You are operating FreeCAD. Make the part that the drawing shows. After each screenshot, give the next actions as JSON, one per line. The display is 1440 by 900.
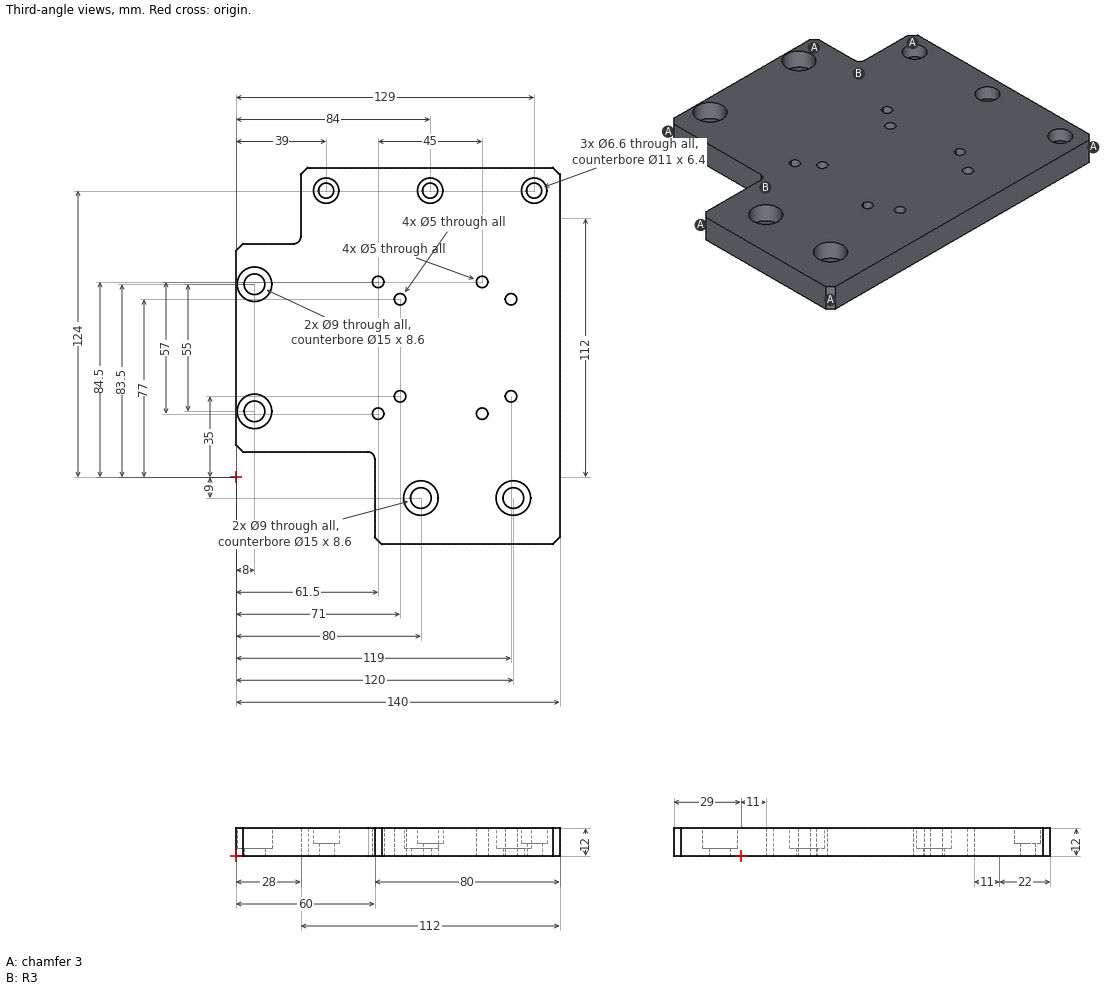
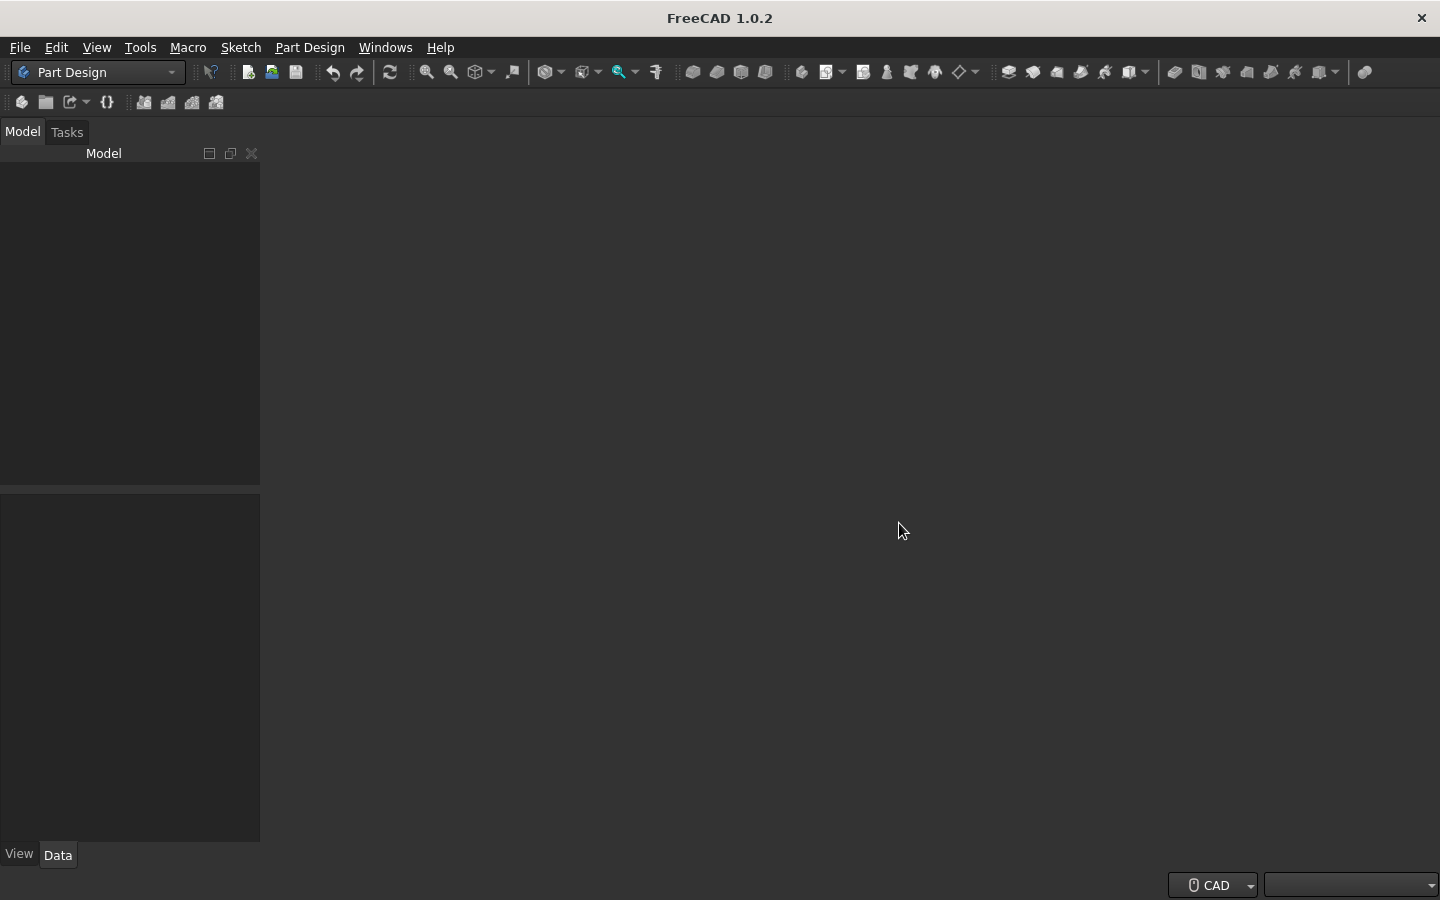
{"action": "left_click", "coordinate": [248, 72]}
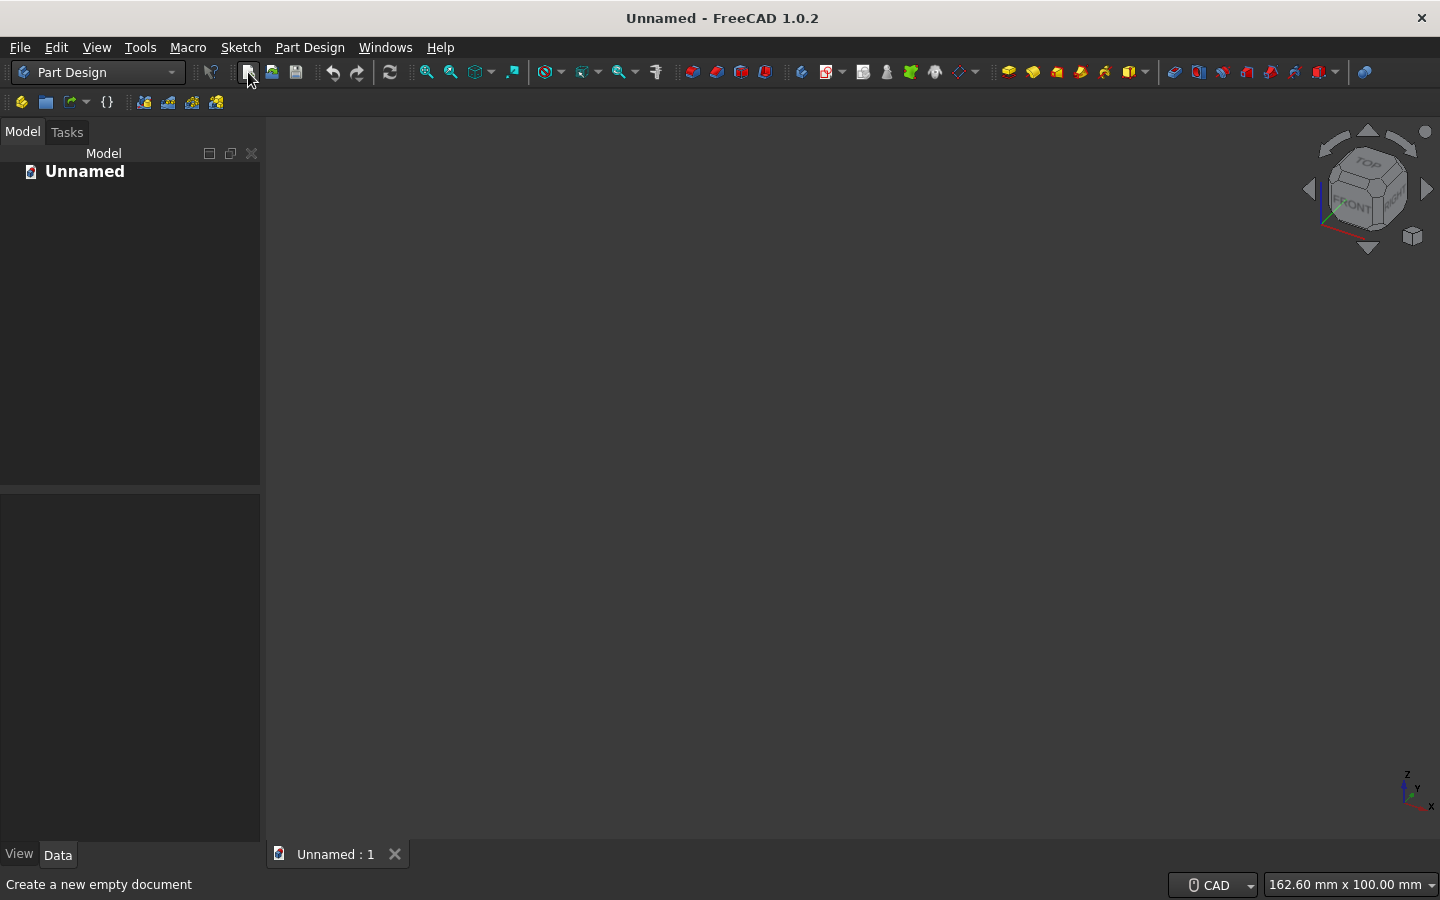
{"action": "left_click", "coordinate": [826, 72]}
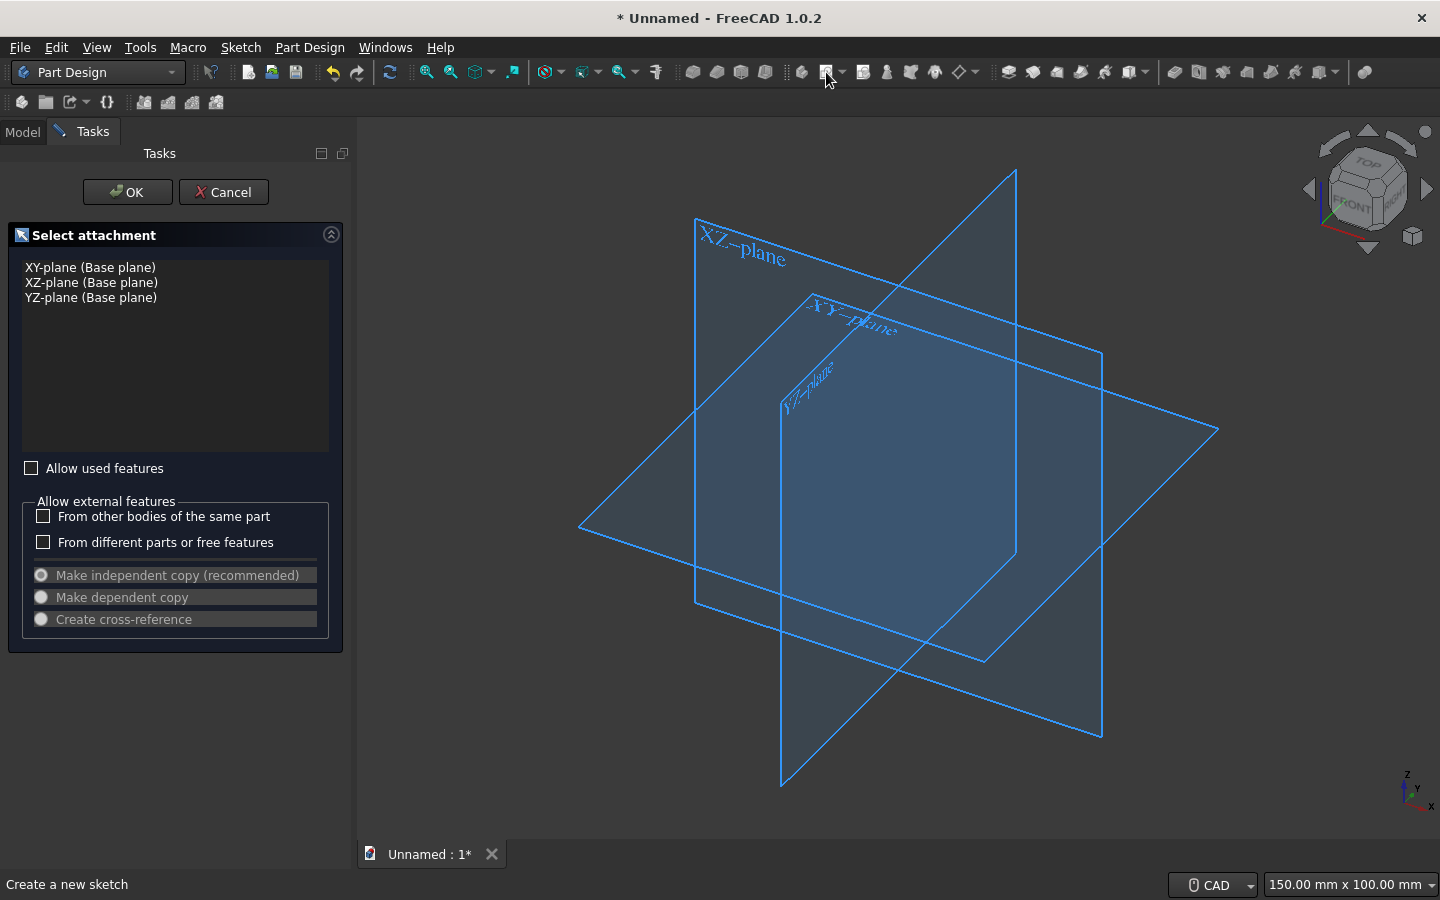
{"action": "left_click", "coordinate": [82, 268]}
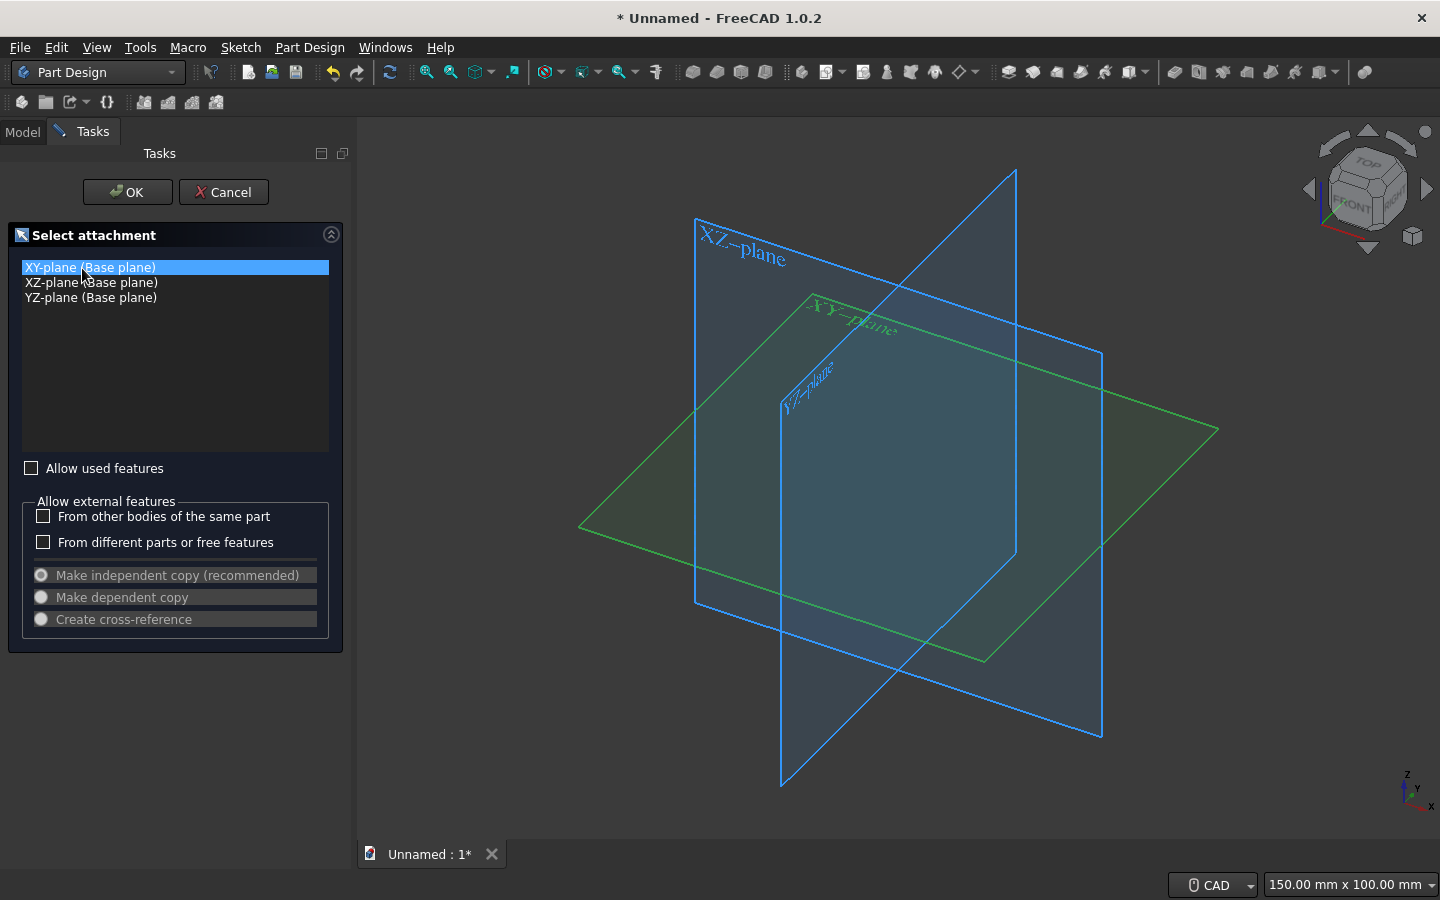
{"action": "left_click", "coordinate": [128, 192]}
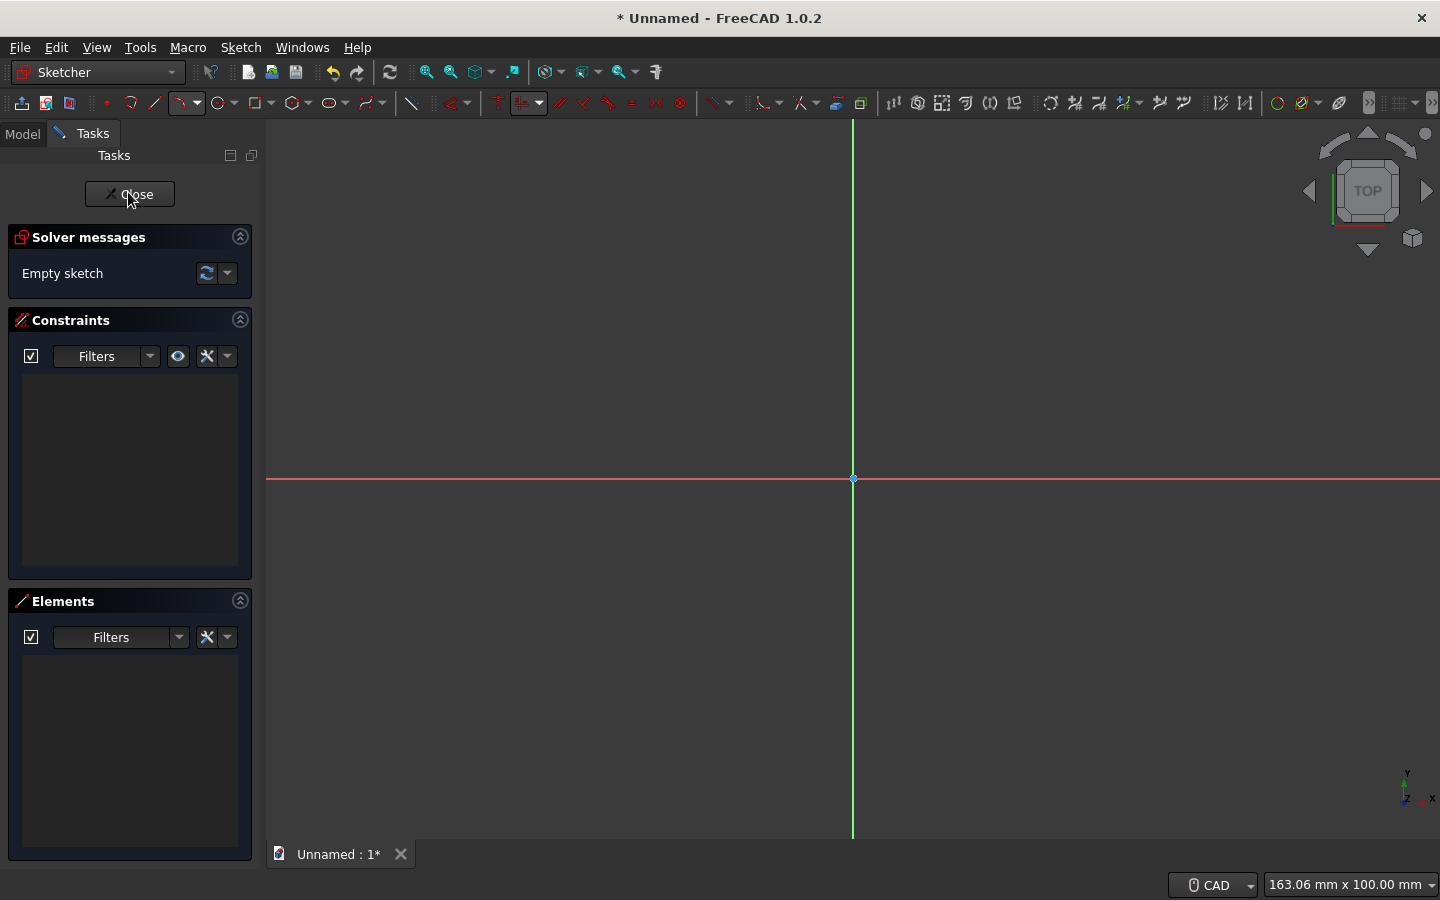
{"action": "scroll", "coordinate": [294, 811], "scroll_direction": "down", "scroll_amount": 3}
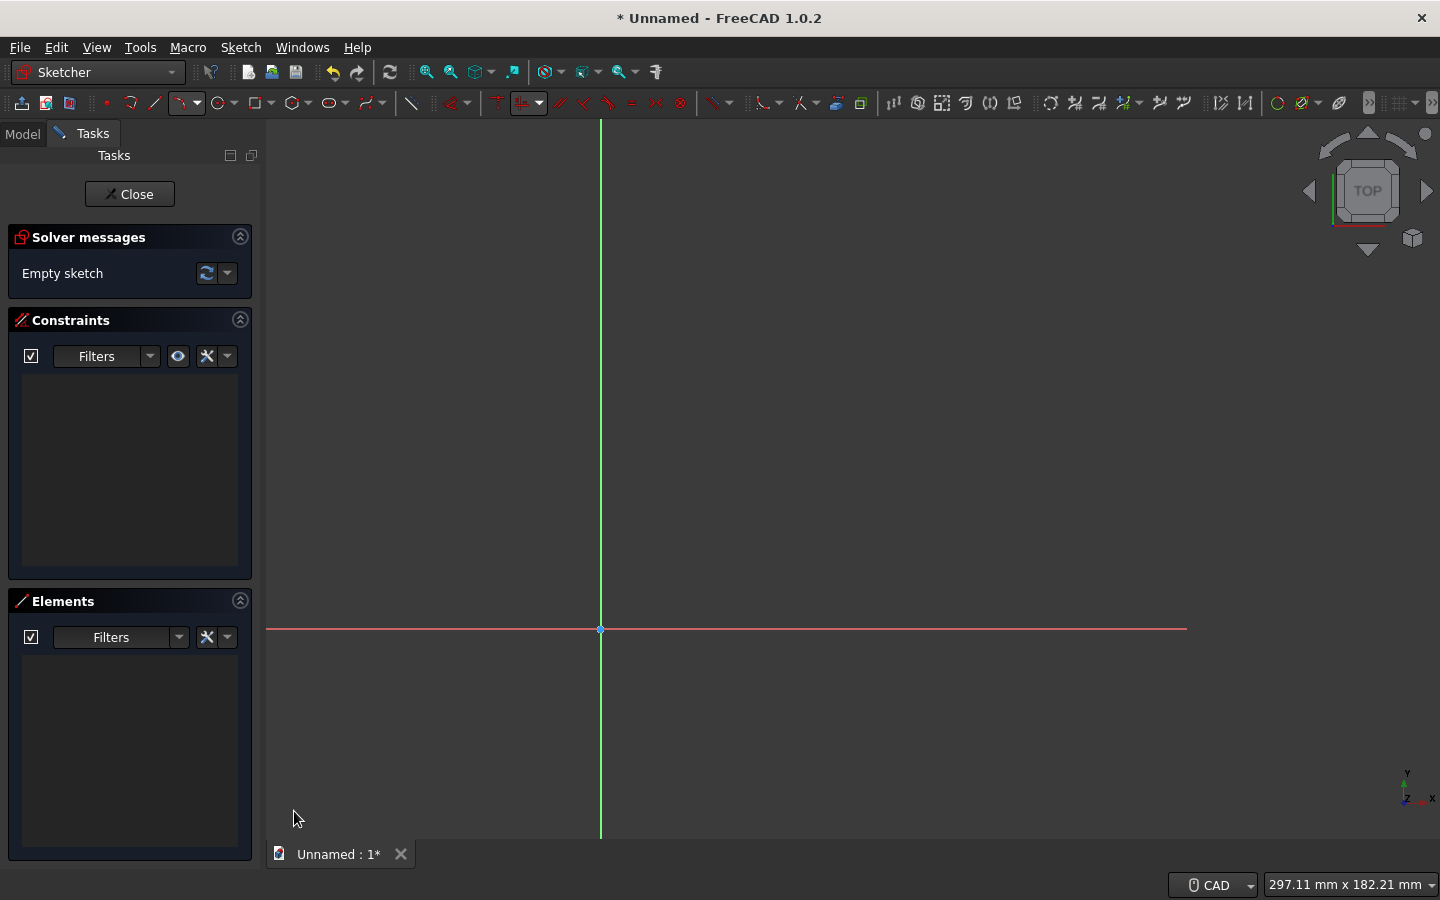
{"action": "left_click", "coordinate": [256, 104]}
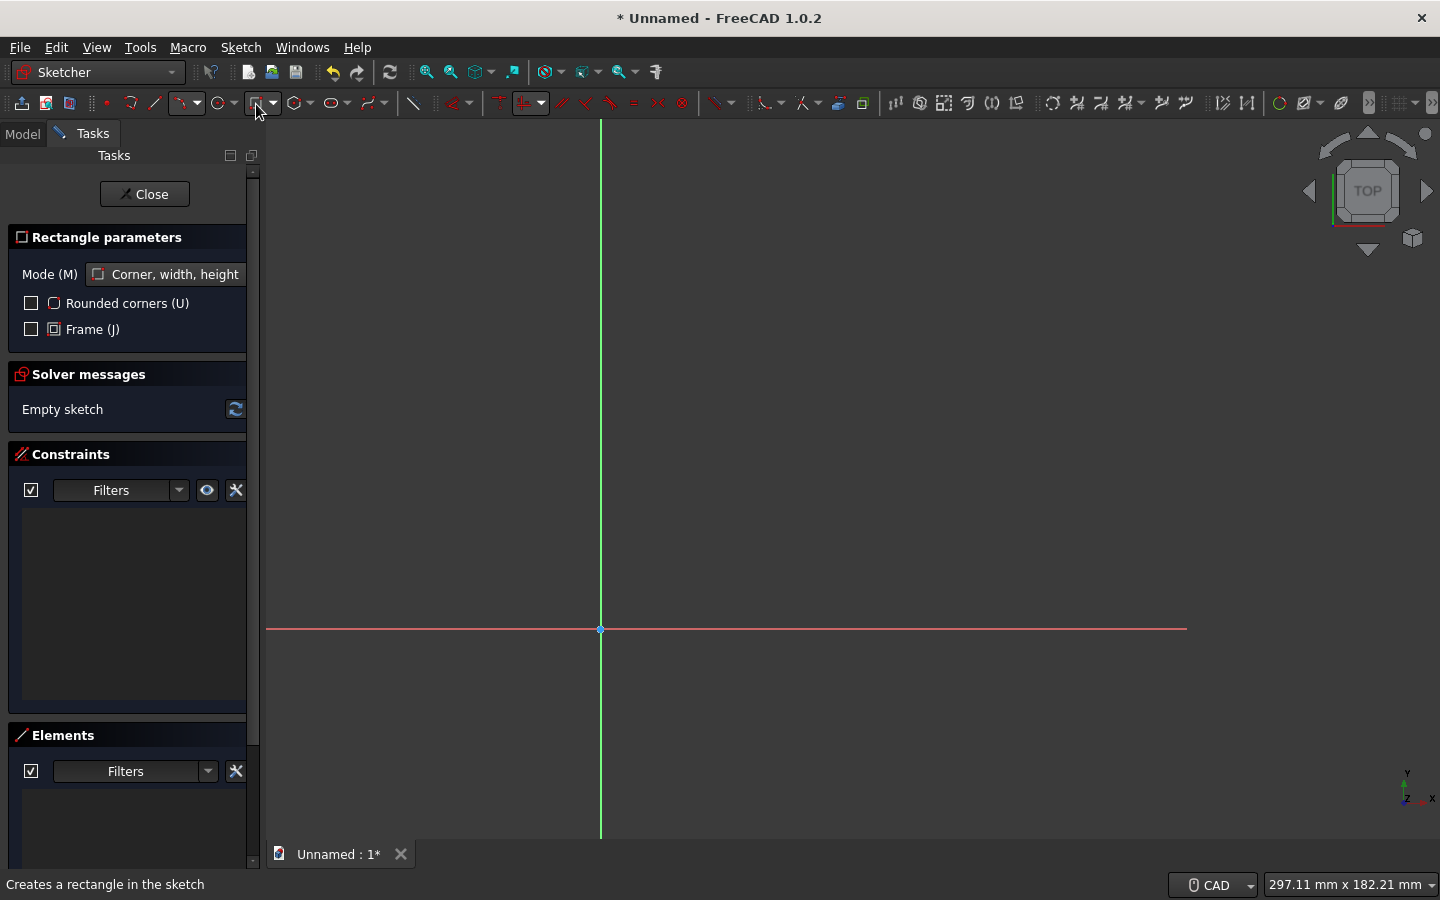
{"action": "left_click", "coordinate": [601, 629]}
{"action": "mouse_move", "coordinate": [1154, 187]}